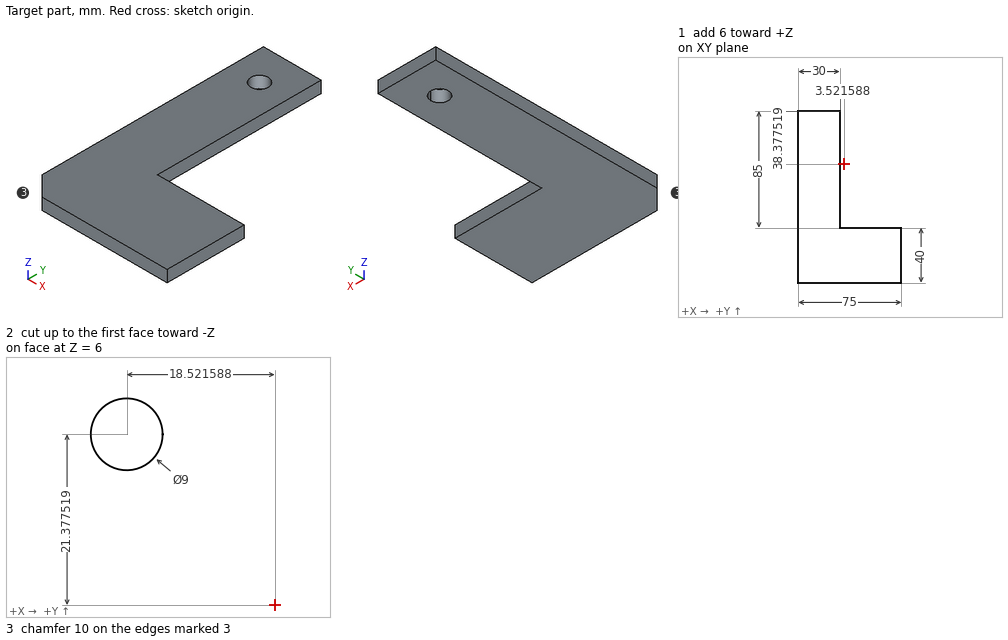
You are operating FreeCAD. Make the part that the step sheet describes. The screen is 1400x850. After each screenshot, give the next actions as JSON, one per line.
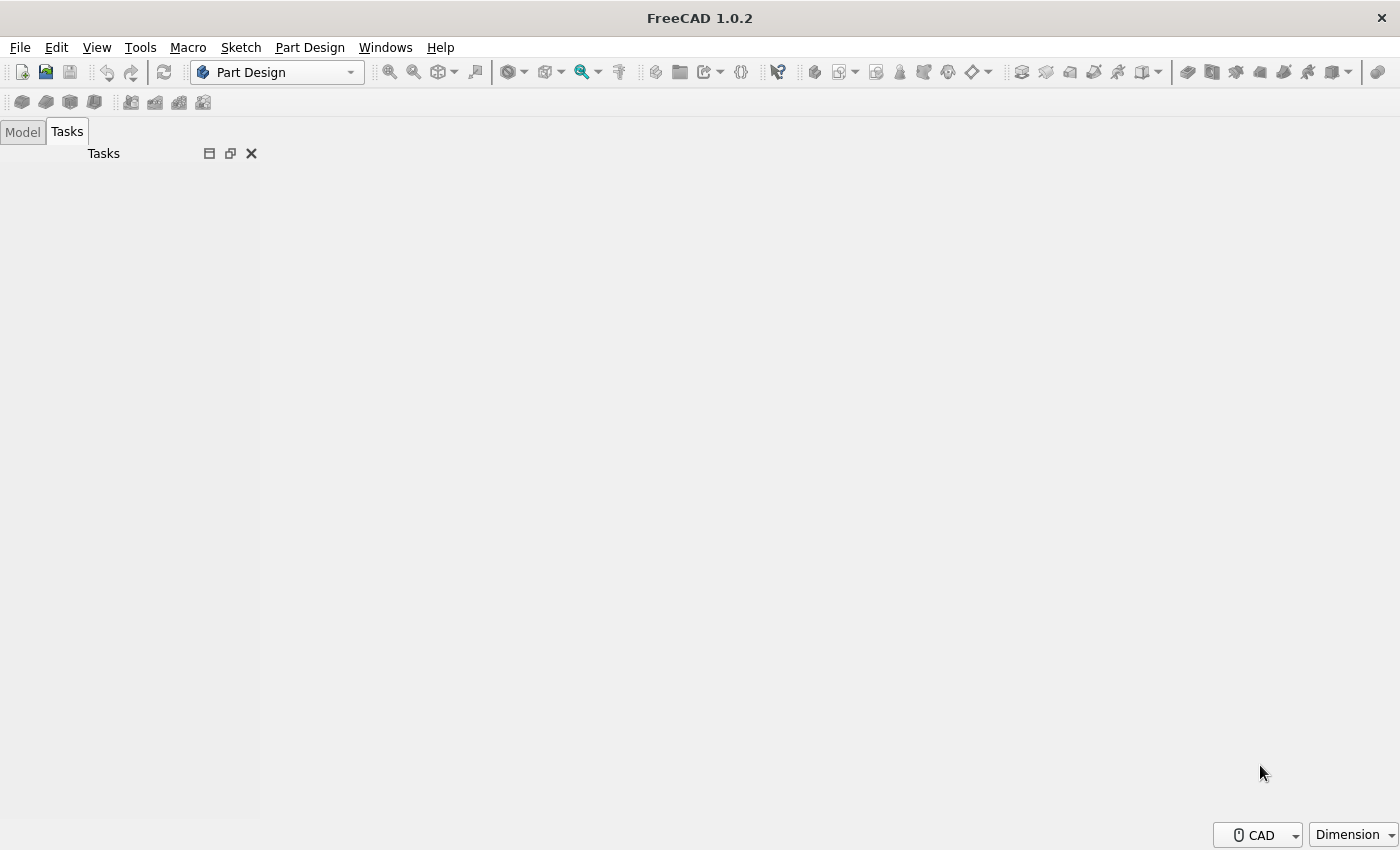
{"action": "left_click", "coordinate": [22, 72]}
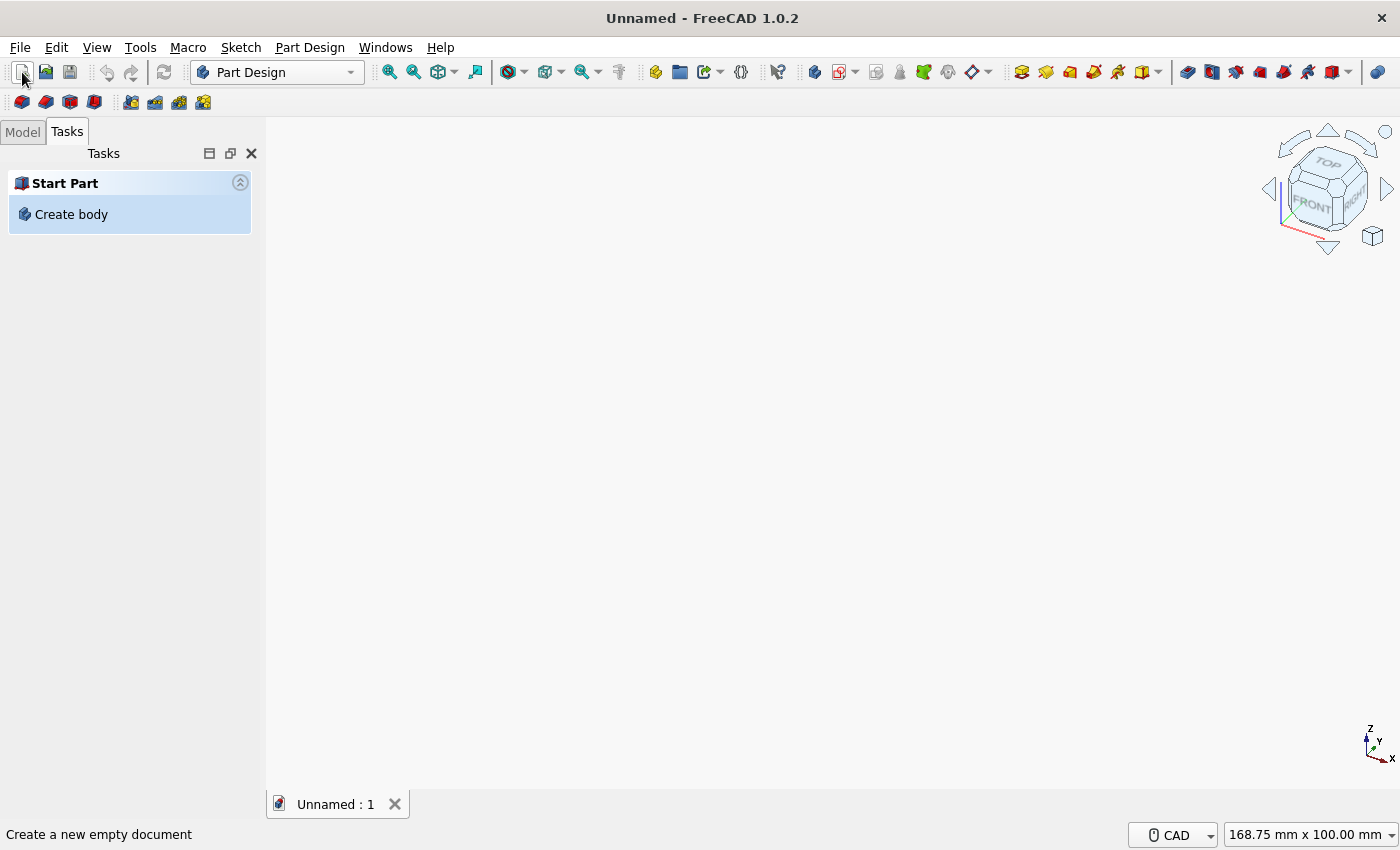
{"action": "left_click", "coordinate": [840, 72]}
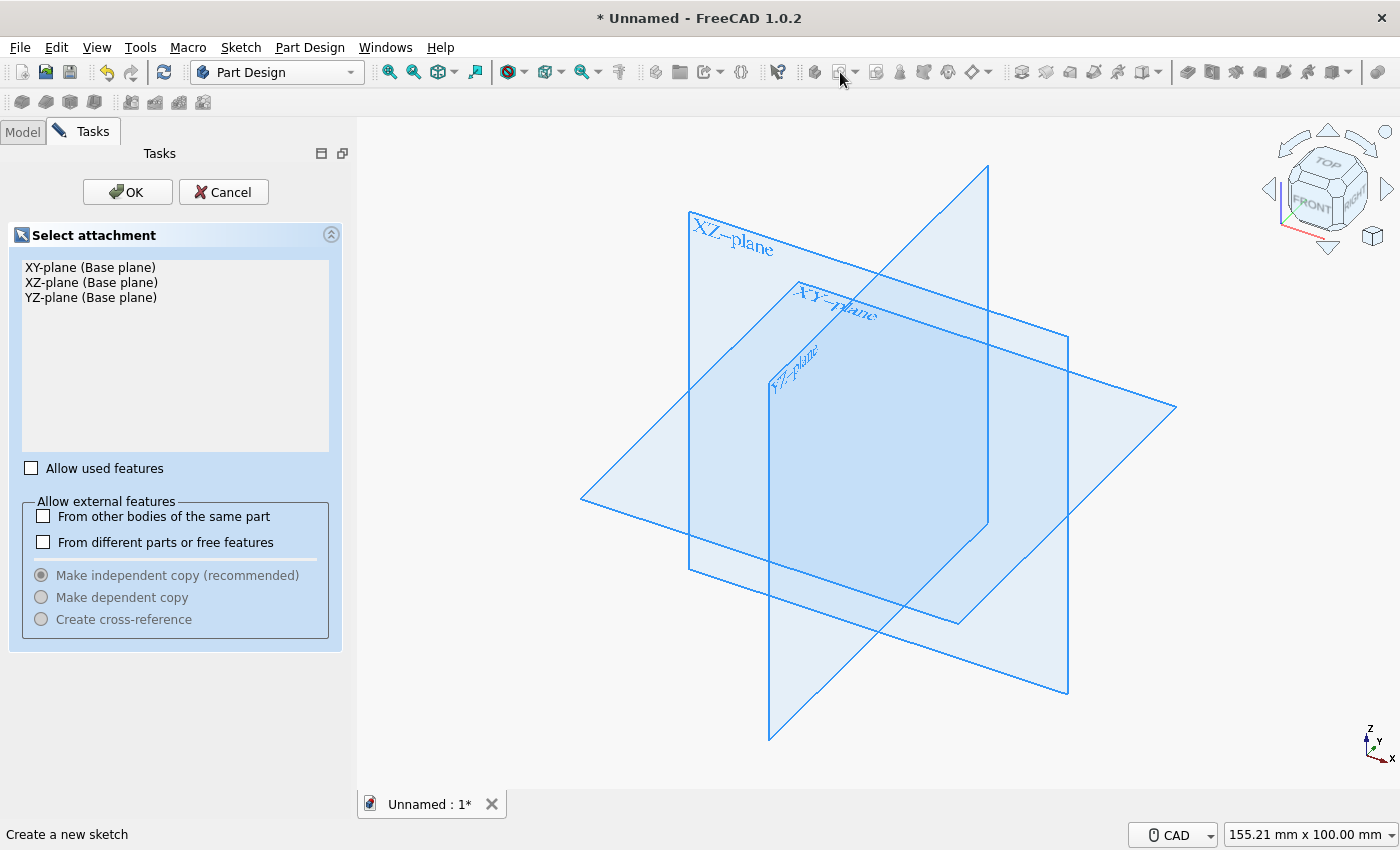
{"action": "left_click", "coordinate": [82, 268]}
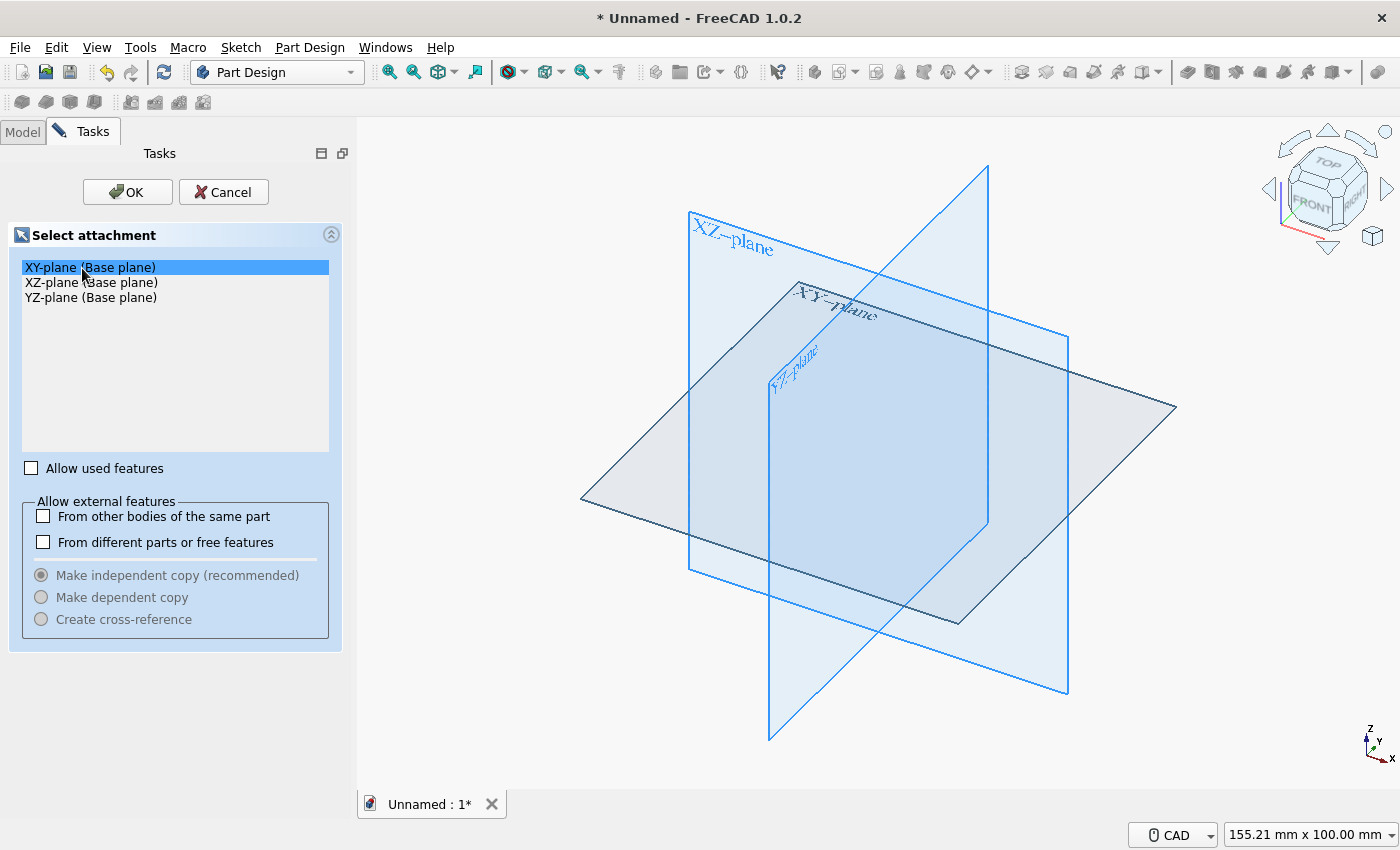
{"action": "left_click", "coordinate": [128, 192]}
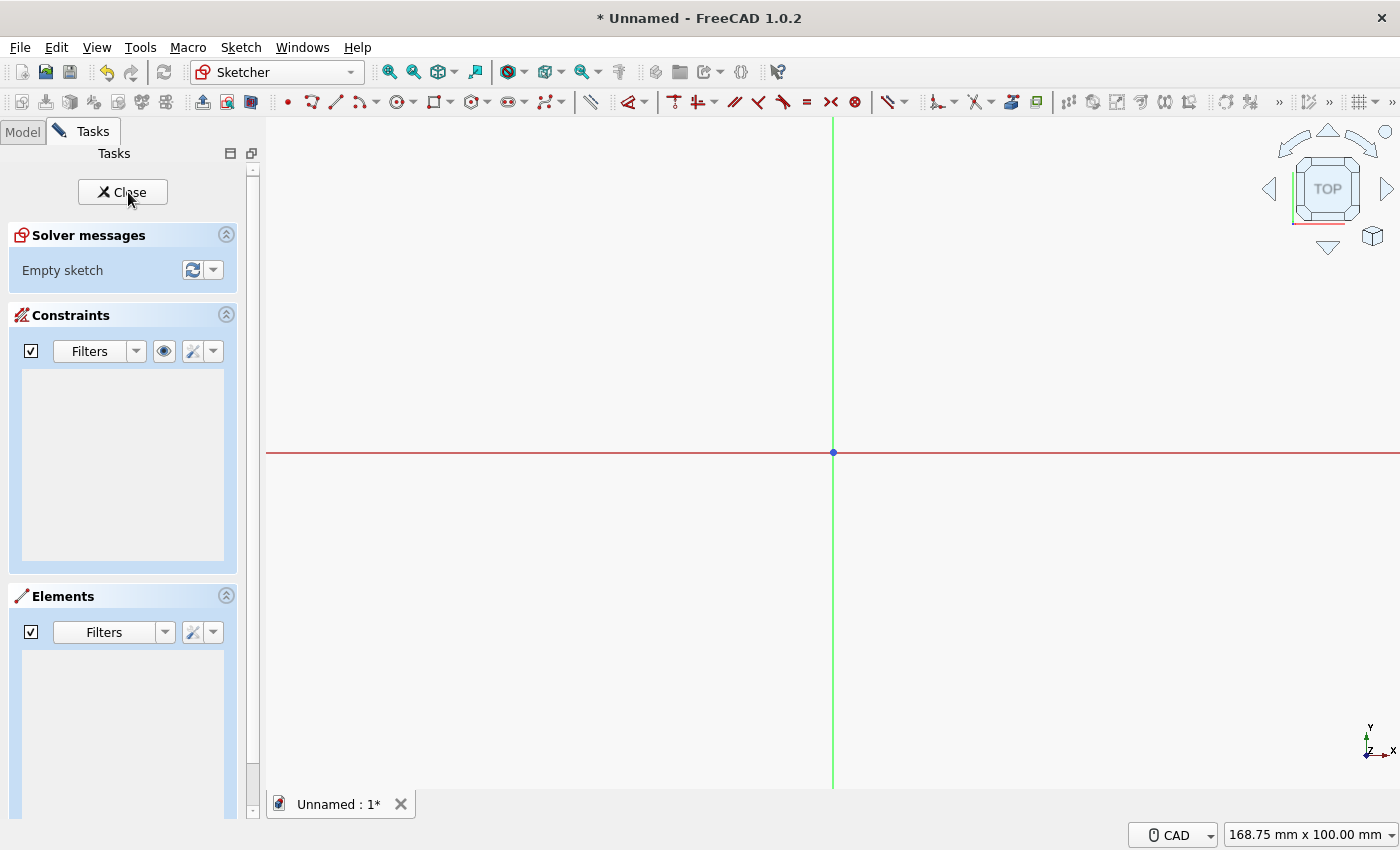
{"action": "scroll", "coordinate": [649, 256], "scroll_direction": "down", "scroll_amount": 3}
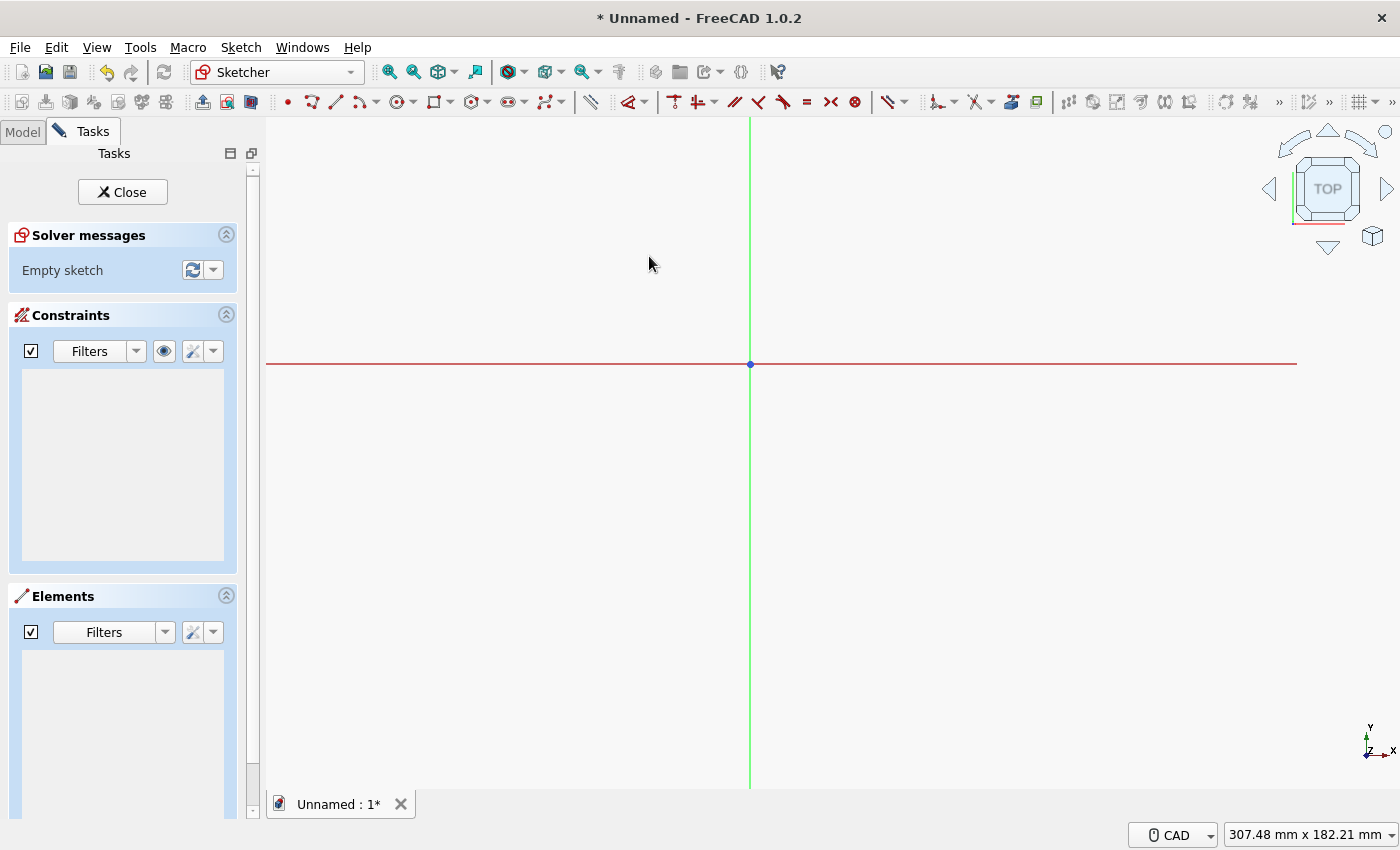
{"action": "left_click", "coordinate": [312, 102]}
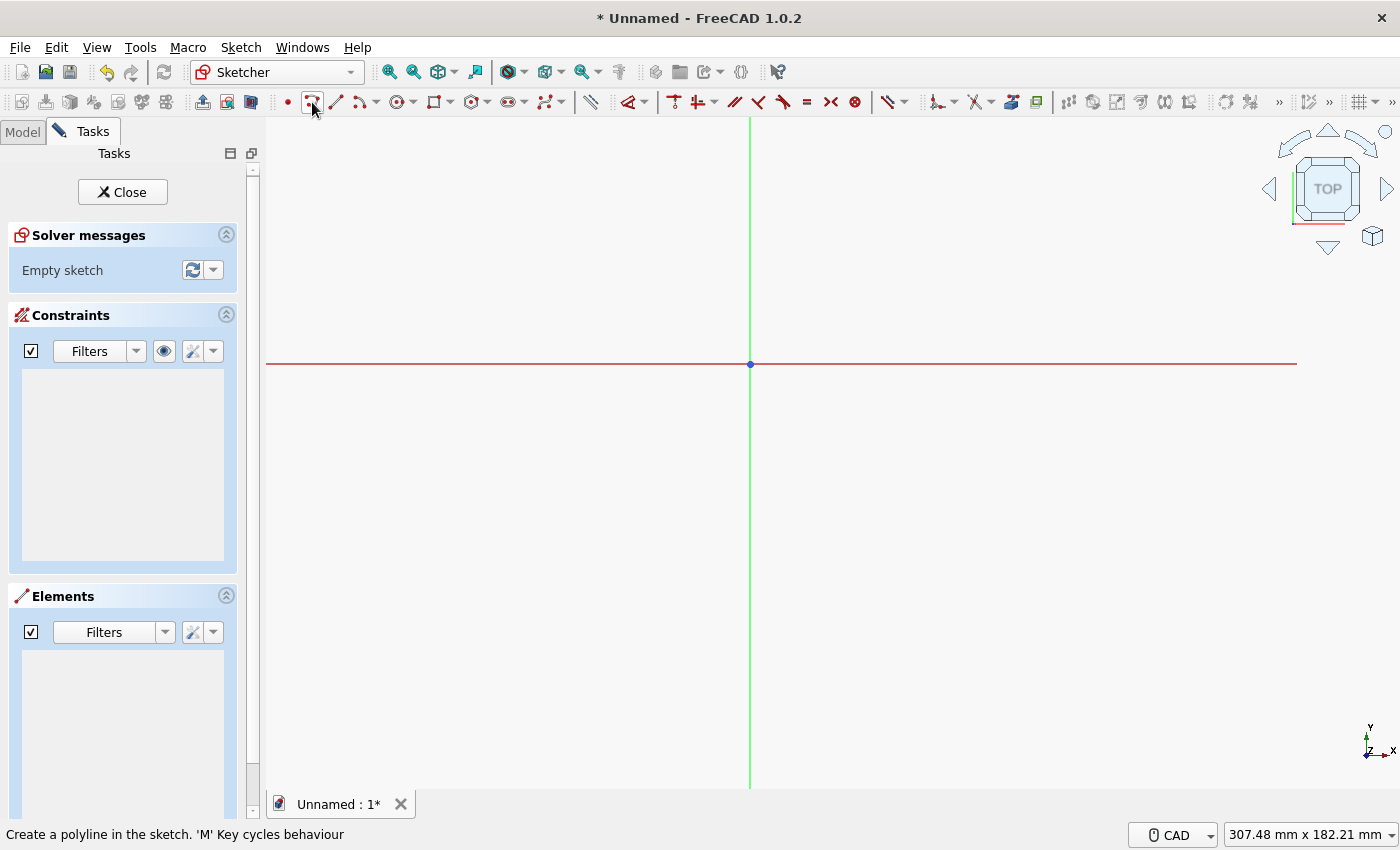
{"action": "scroll", "coordinate": [737, 223], "scroll_direction": "up", "scroll_amount": 2}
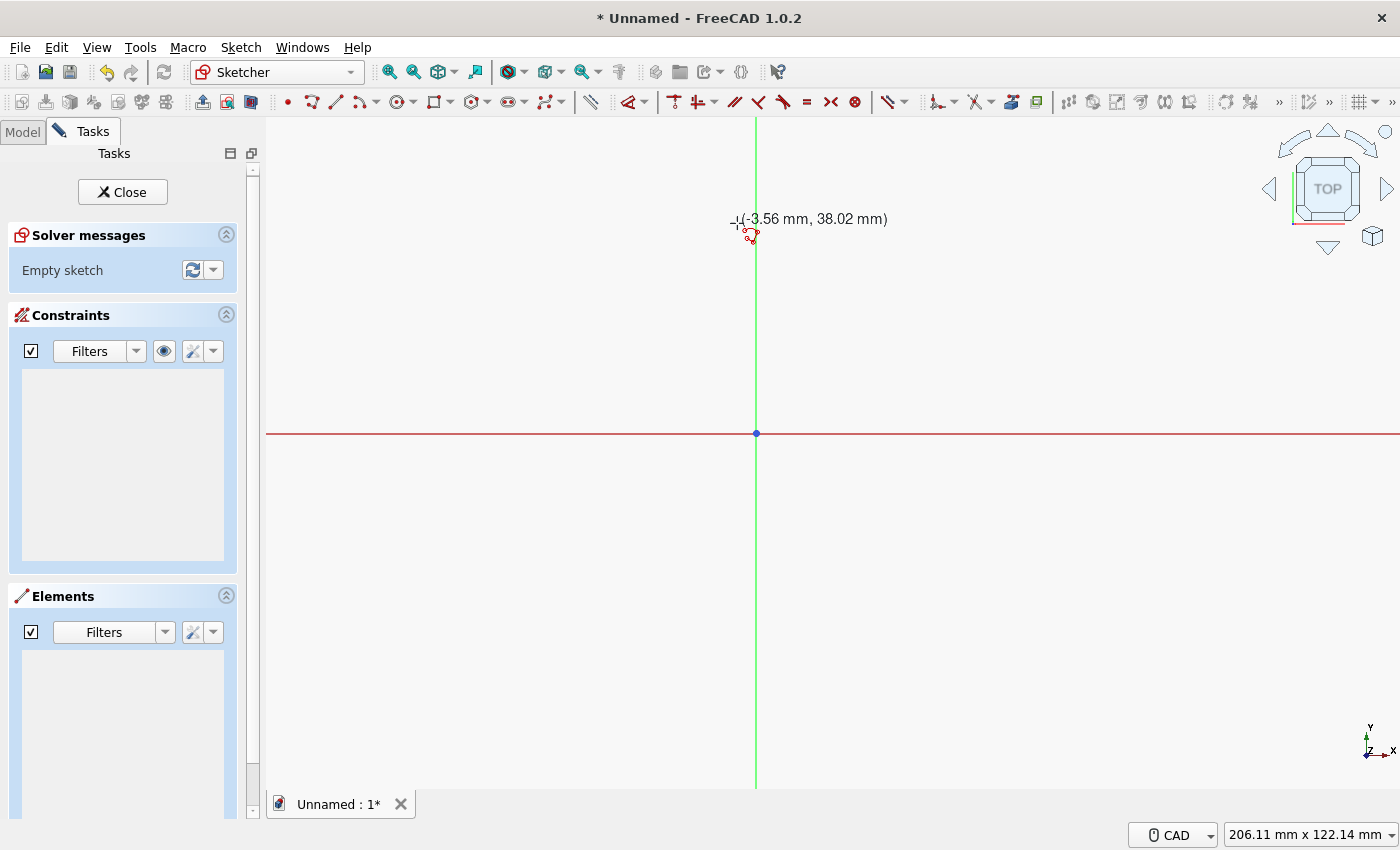
{"action": "left_click", "coordinate": [737, 222]}
{"action": "left_click", "coordinate": [572, 222]}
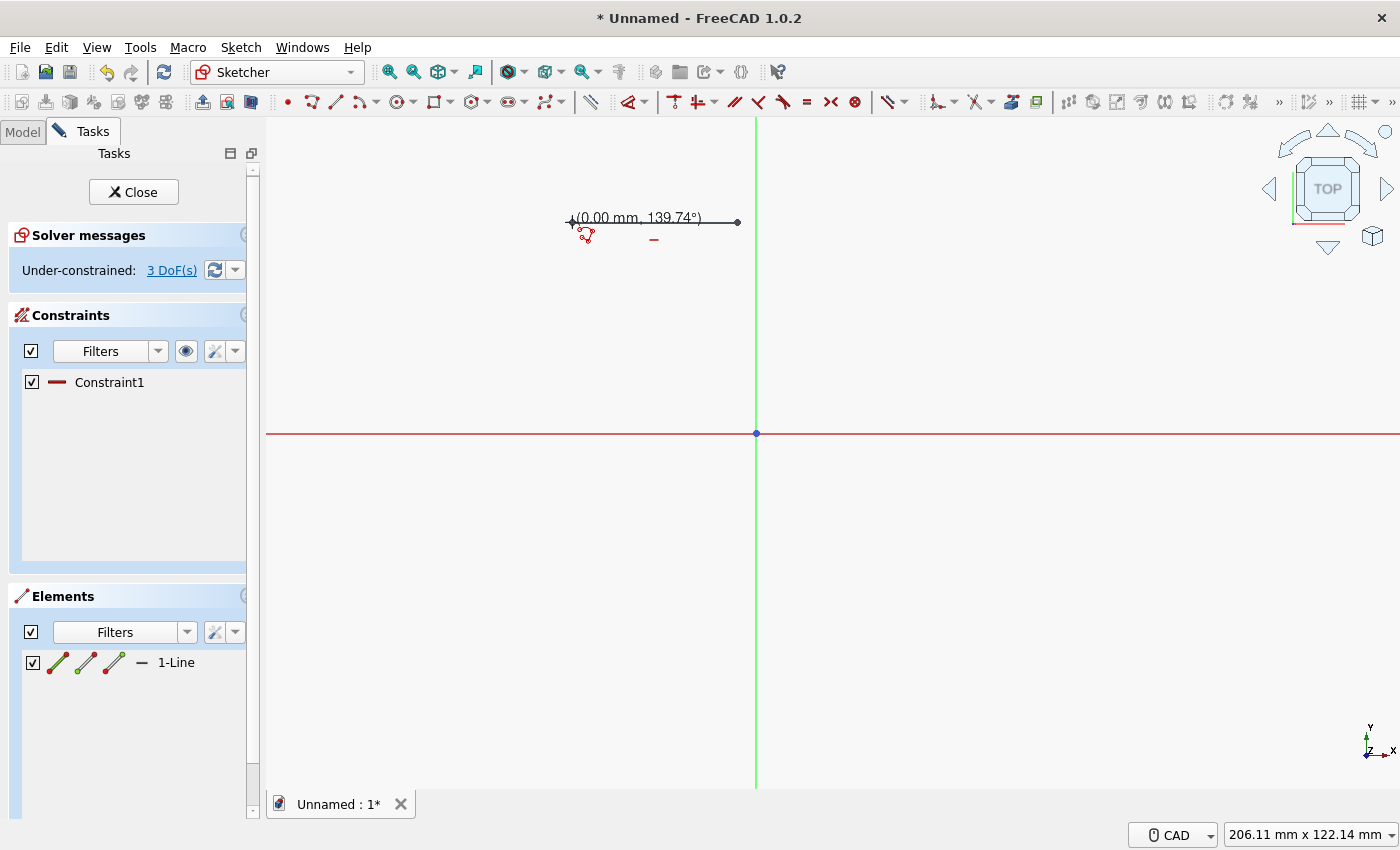
{"action": "scroll", "coordinate": [736, 223], "scroll_direction": "down", "scroll_amount": 2}